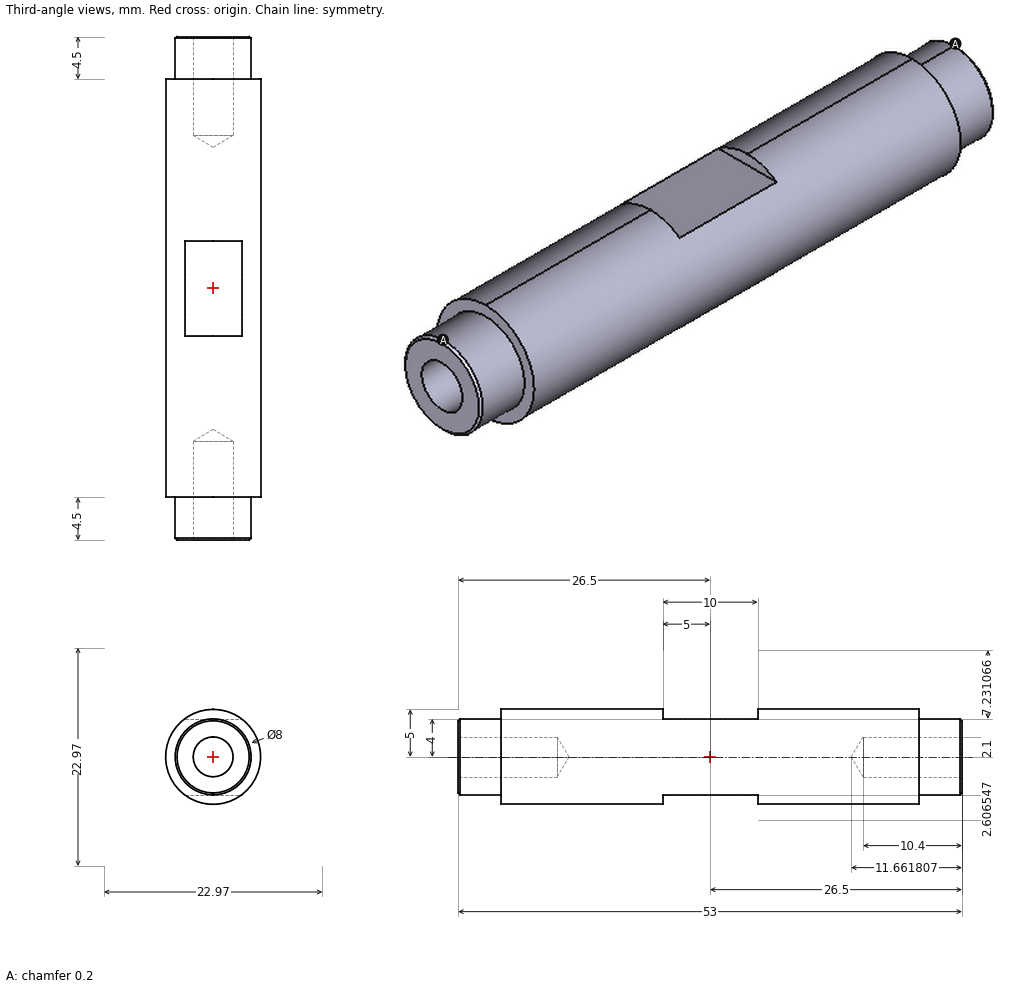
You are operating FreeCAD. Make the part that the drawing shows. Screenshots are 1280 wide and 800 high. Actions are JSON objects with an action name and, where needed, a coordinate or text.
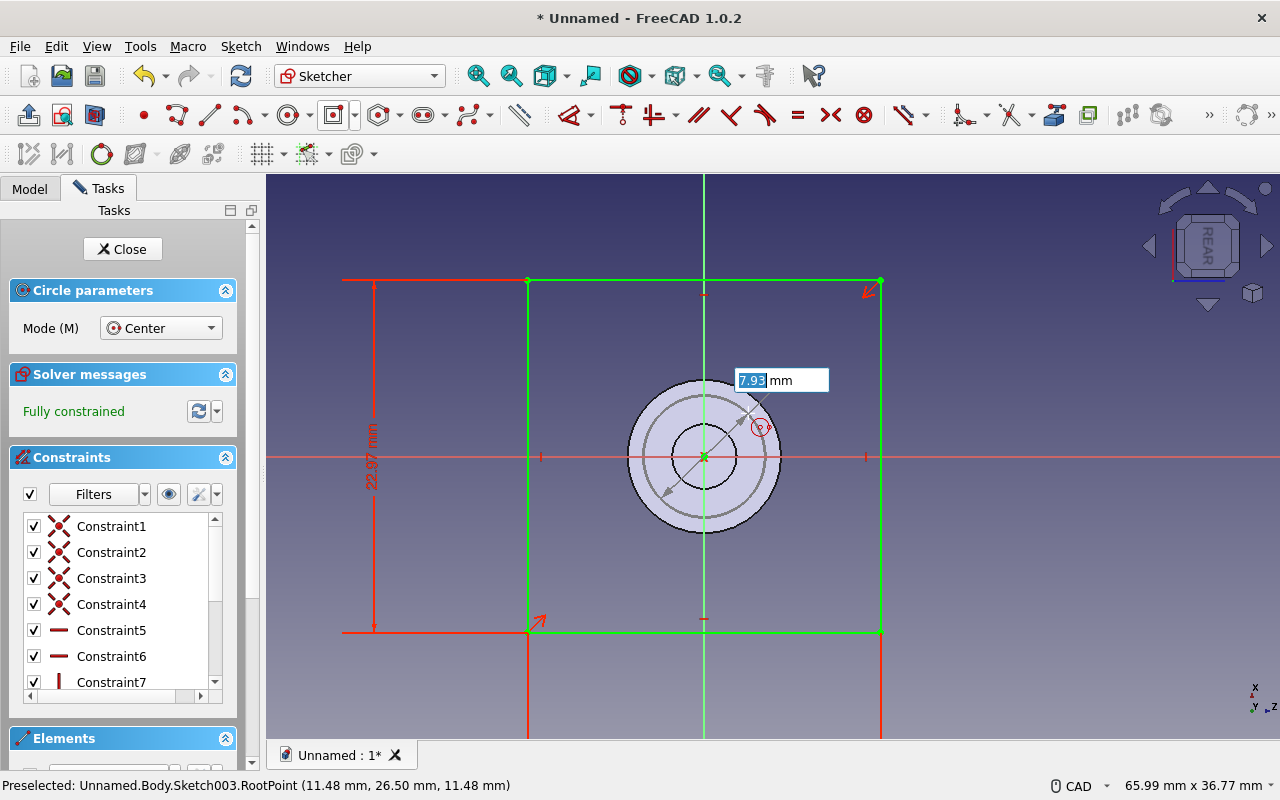
{"action": "type", "text": "8"}
{"action": "key", "text": "Return"}
{"action": "key", "text": "Escape"}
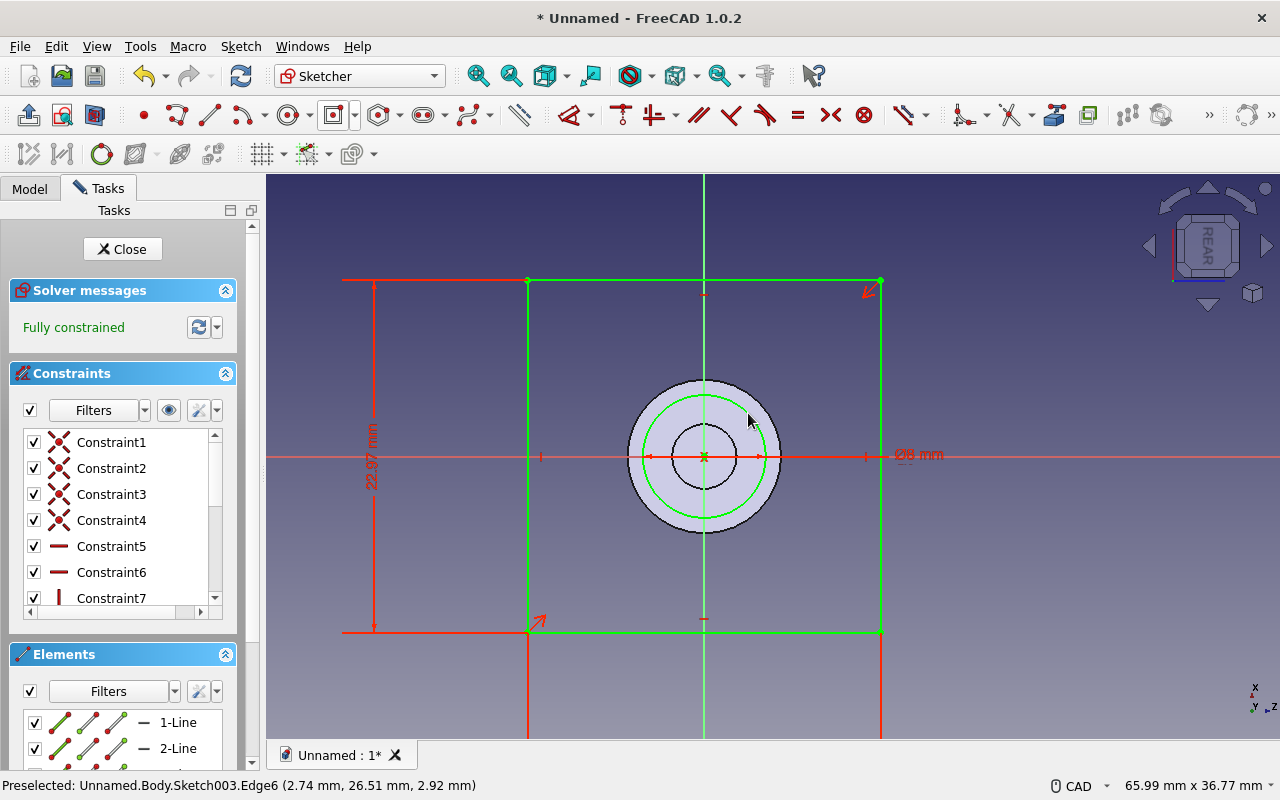
{"action": "left_click", "coordinate": [123, 249]}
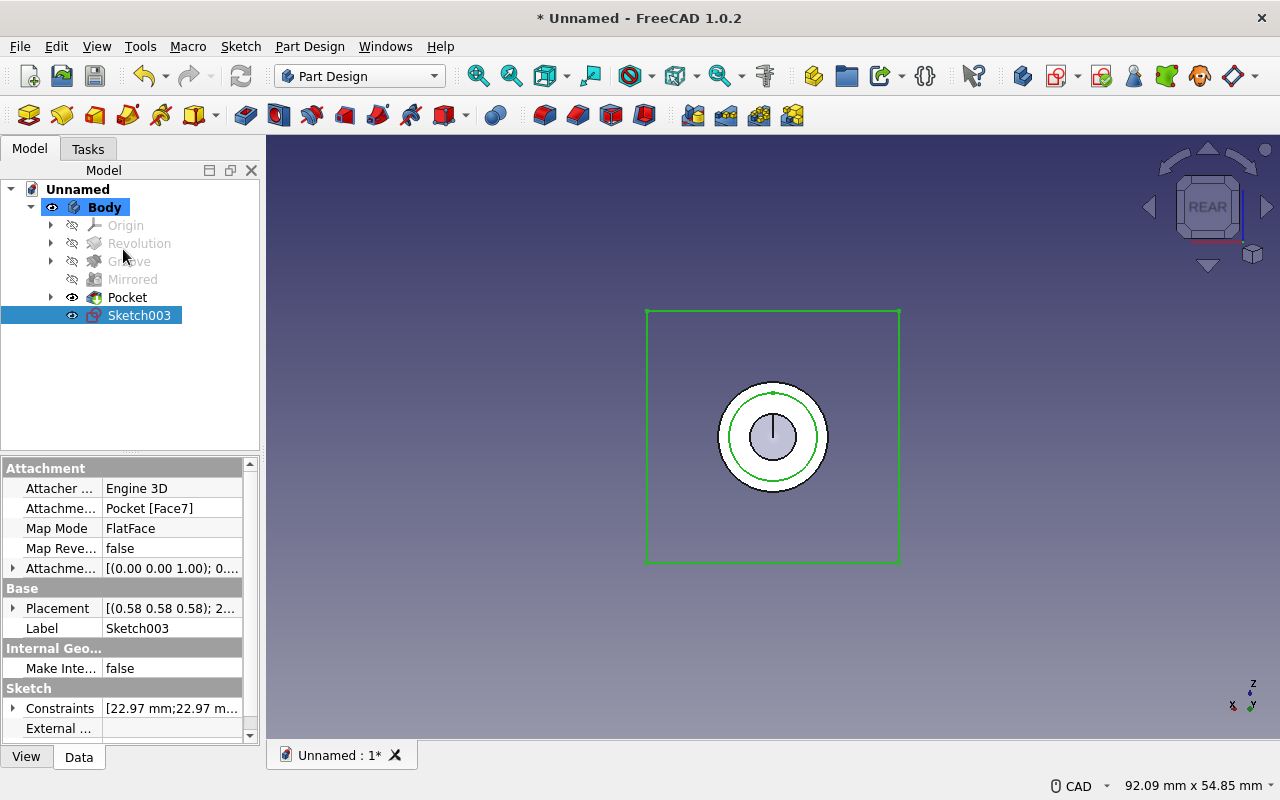
{"action": "left_click", "coordinate": [246, 116]}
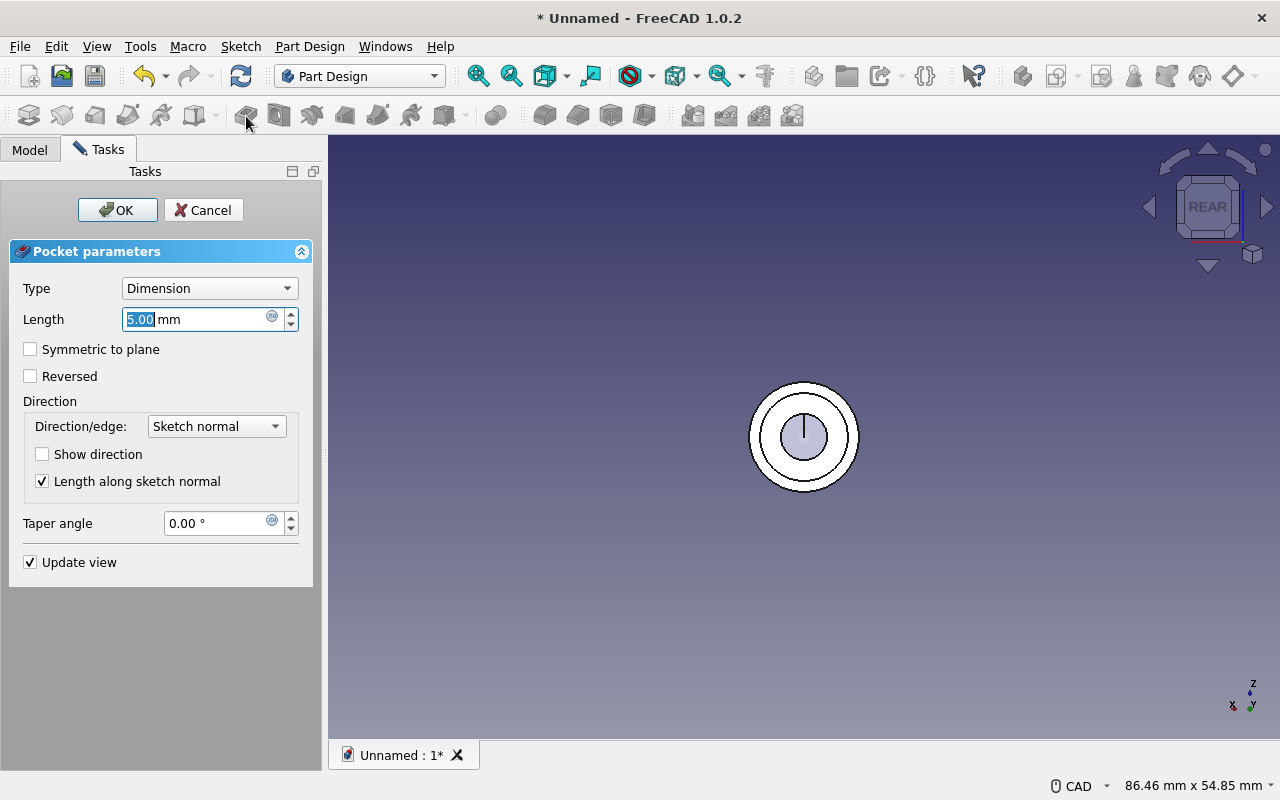
{"action": "type", "text": "4.5"}
{"action": "key", "text": "Tab"}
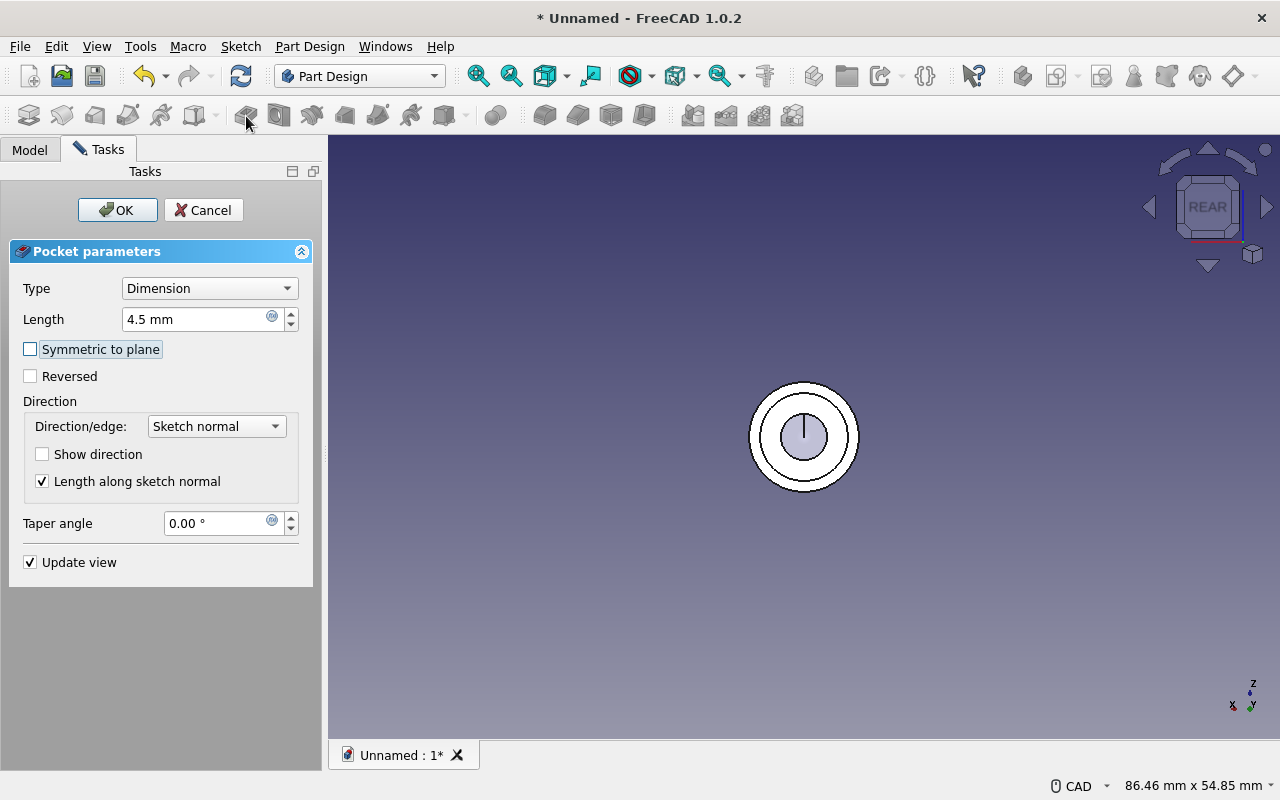
{"action": "left_click", "coordinate": [118, 210]}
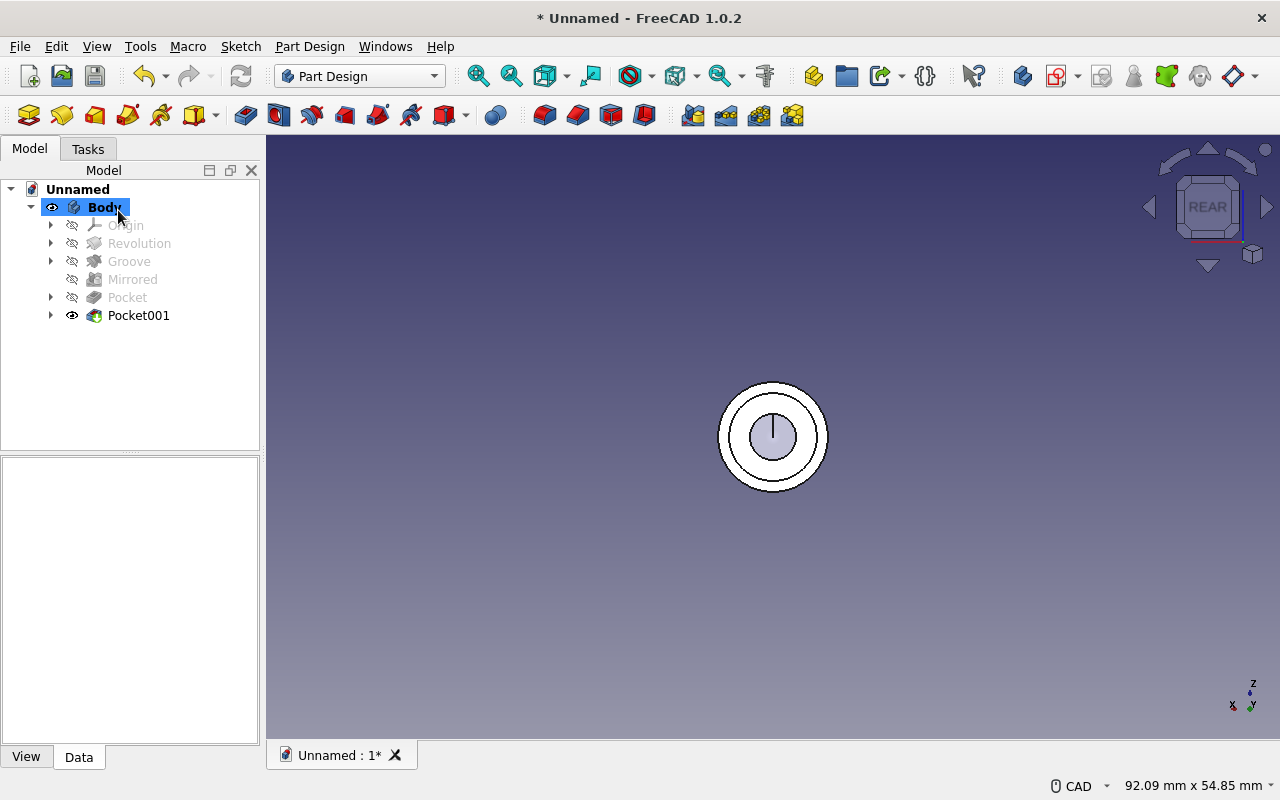
{"action": "left_click", "coordinate": [479, 76]}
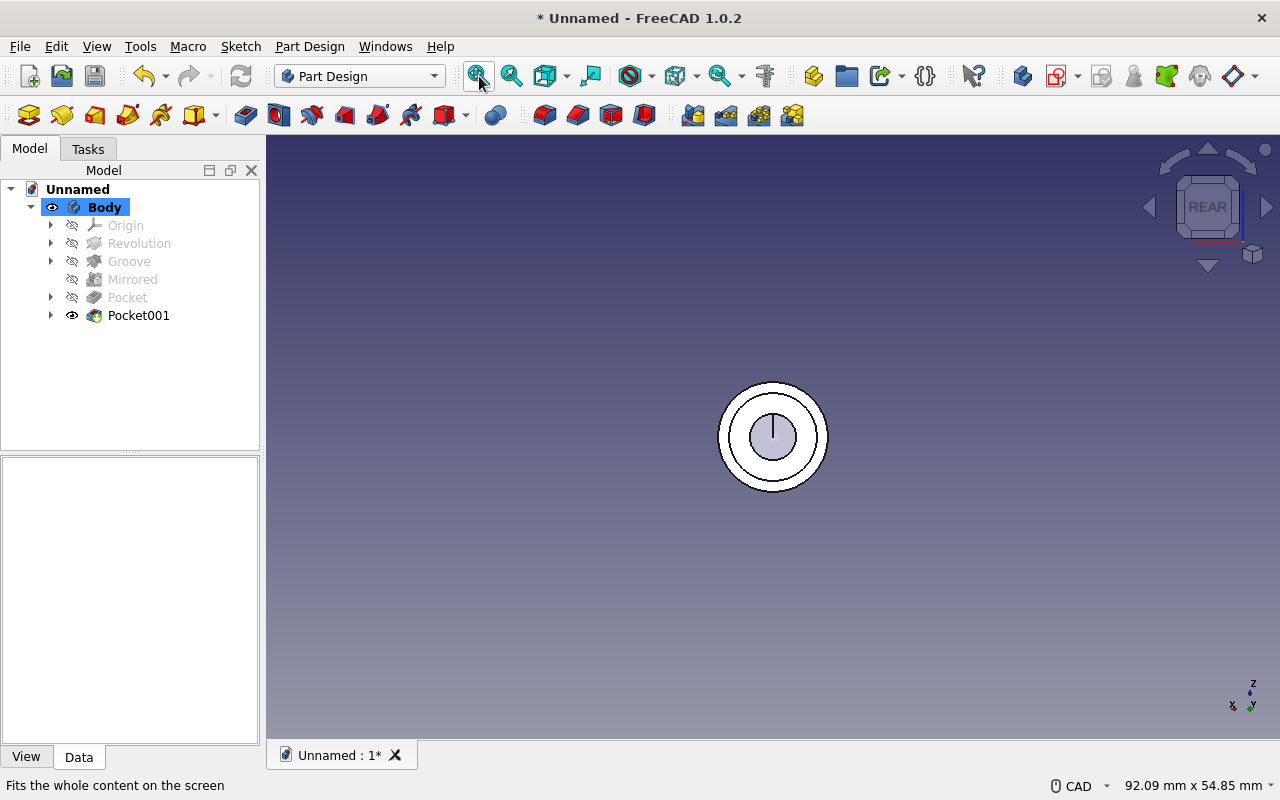
{"action": "left_click", "coordinate": [1056, 76]}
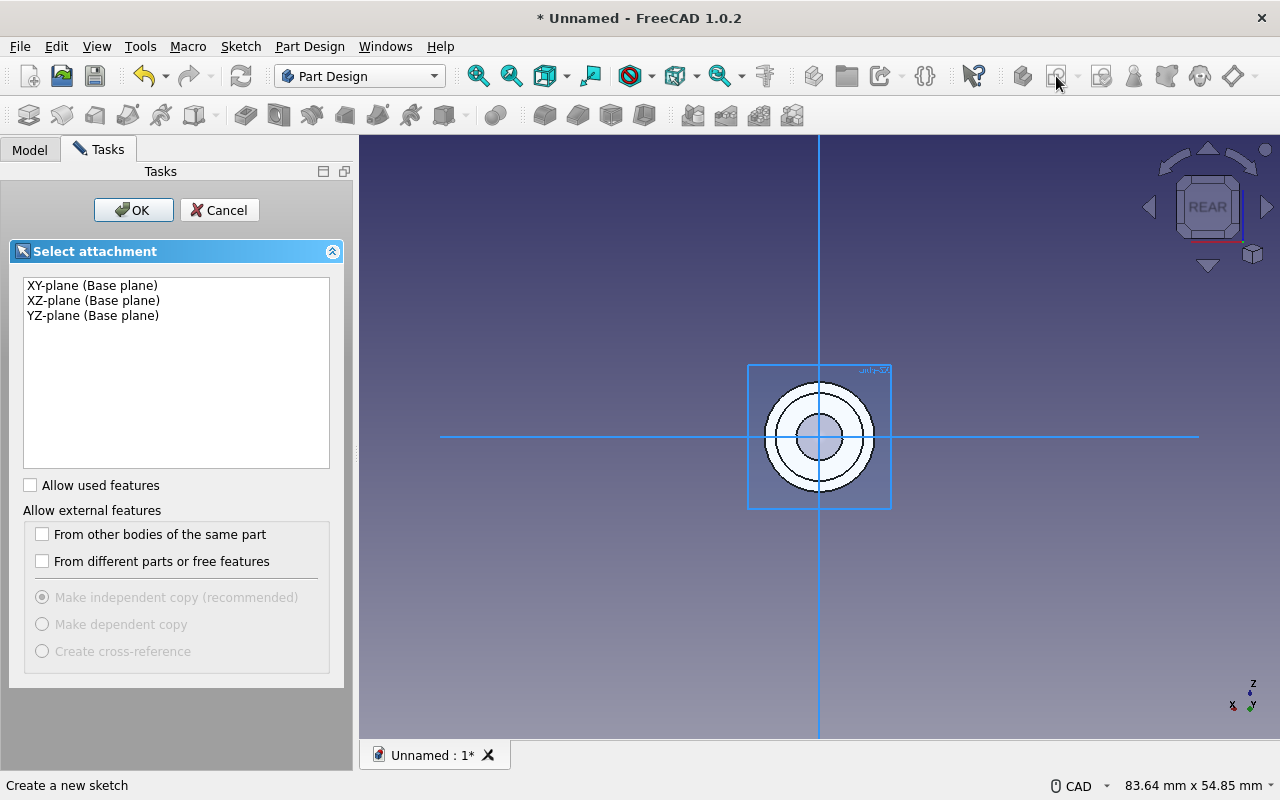
{"action": "left_click", "coordinate": [84, 316]}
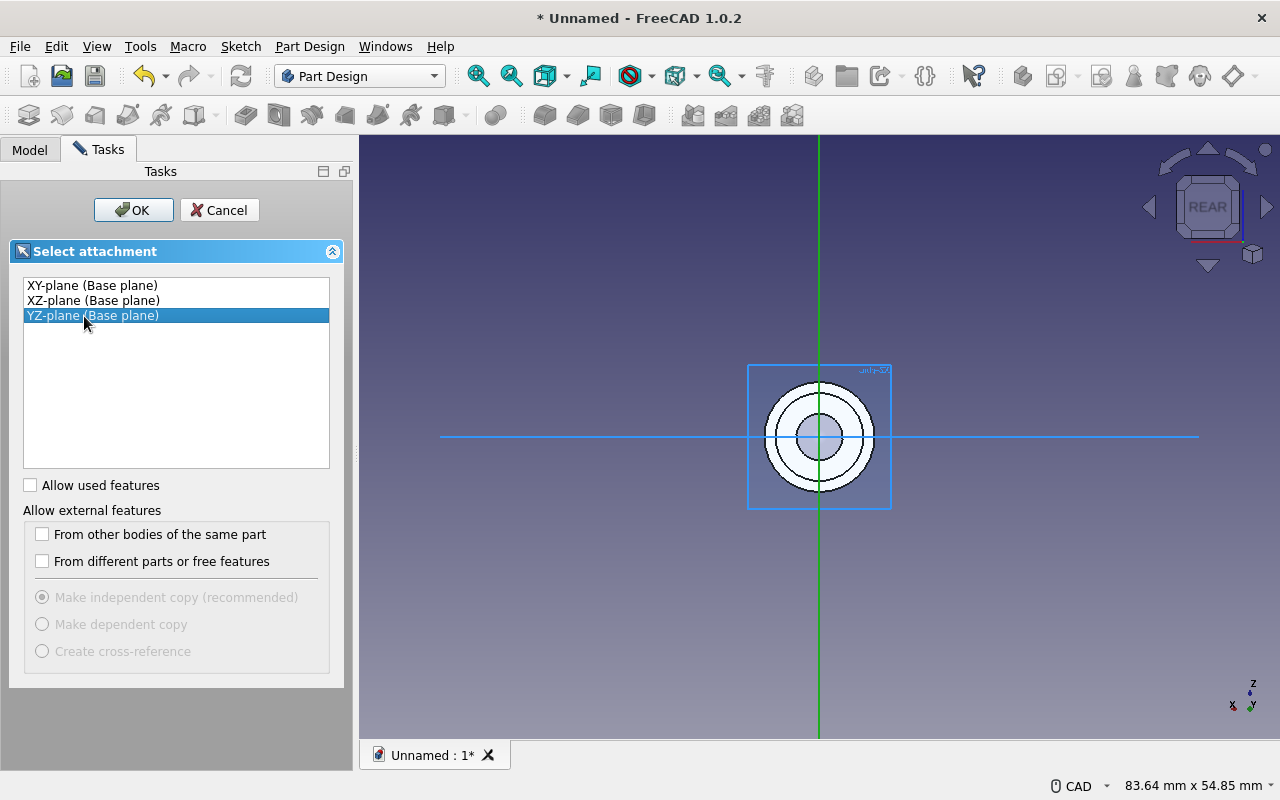
{"action": "left_click", "coordinate": [134, 210]}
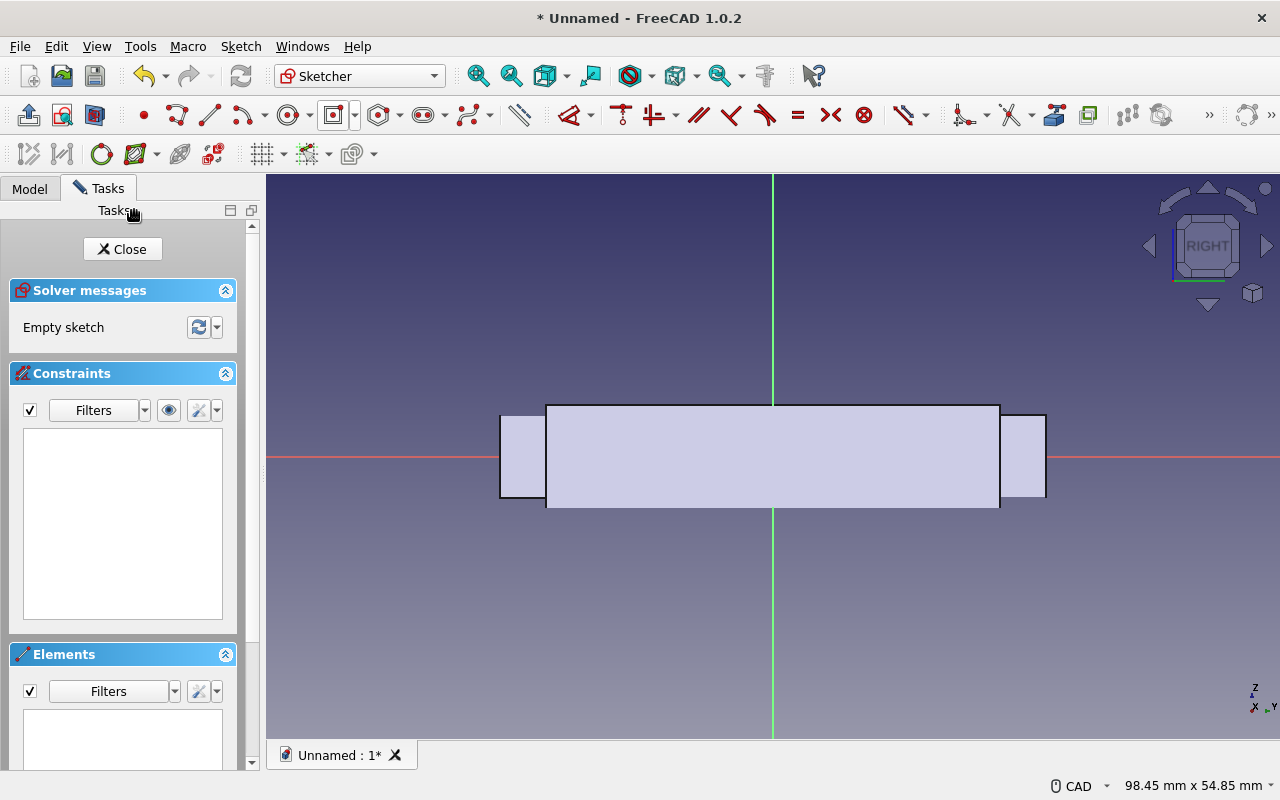
{"action": "left_click", "coordinate": [95, 116]}